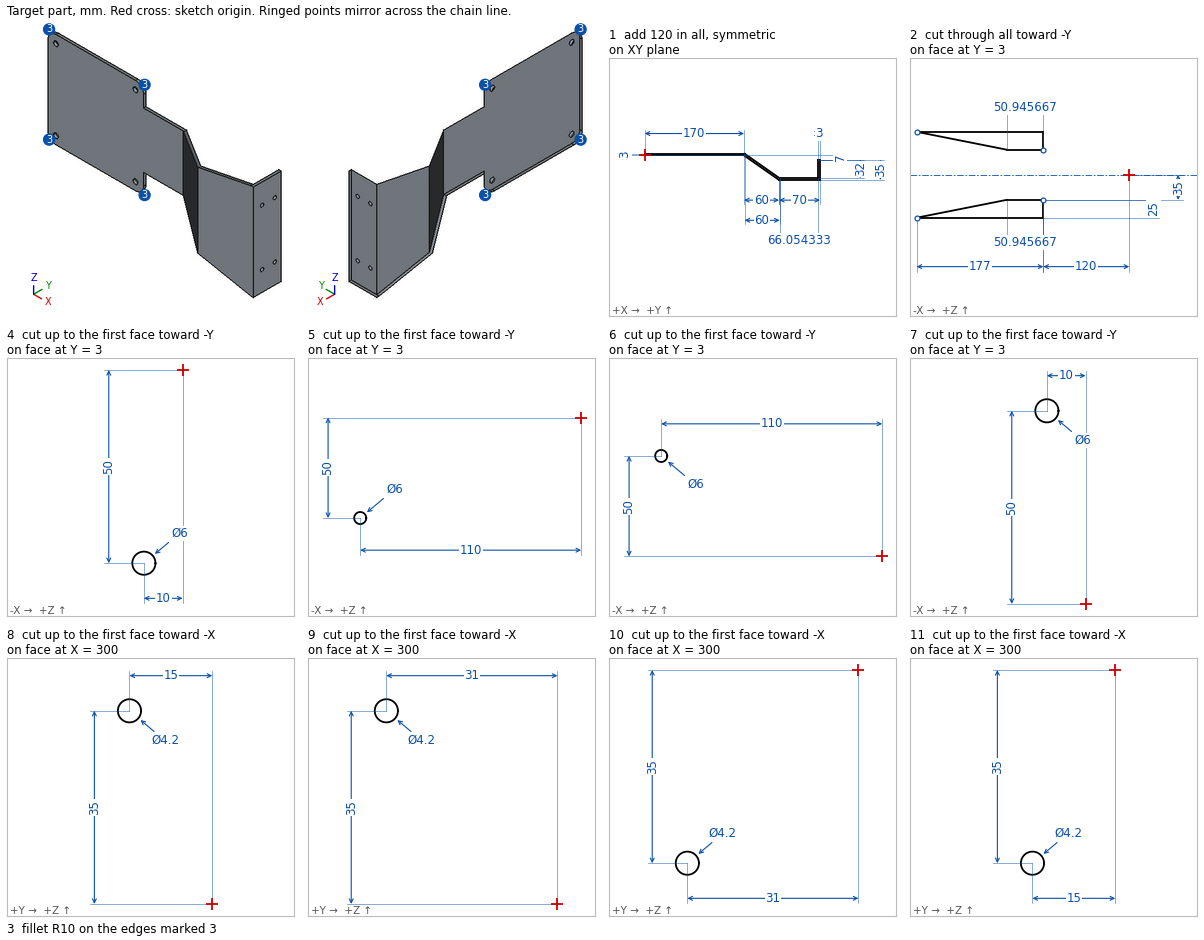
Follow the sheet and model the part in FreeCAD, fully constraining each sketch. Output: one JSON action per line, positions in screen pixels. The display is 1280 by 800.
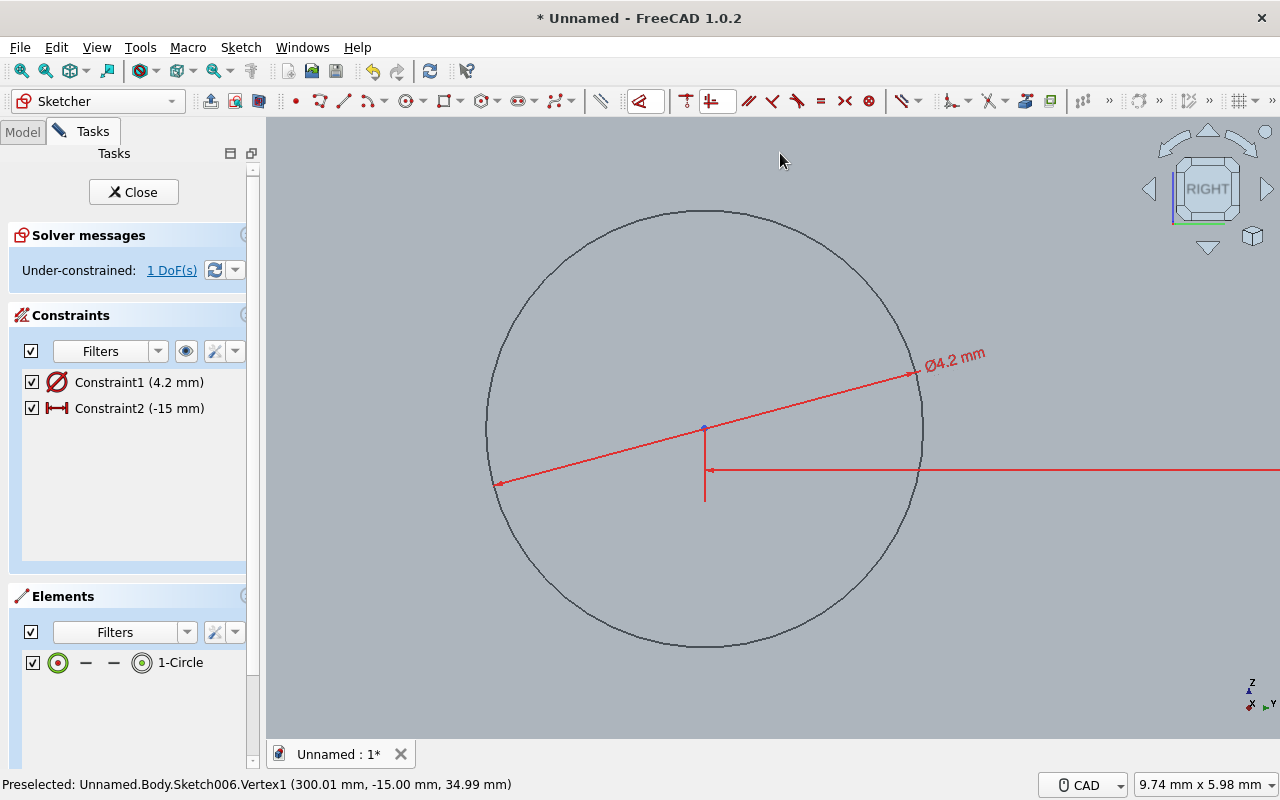
{"action": "left_click", "coordinate": [705, 429]}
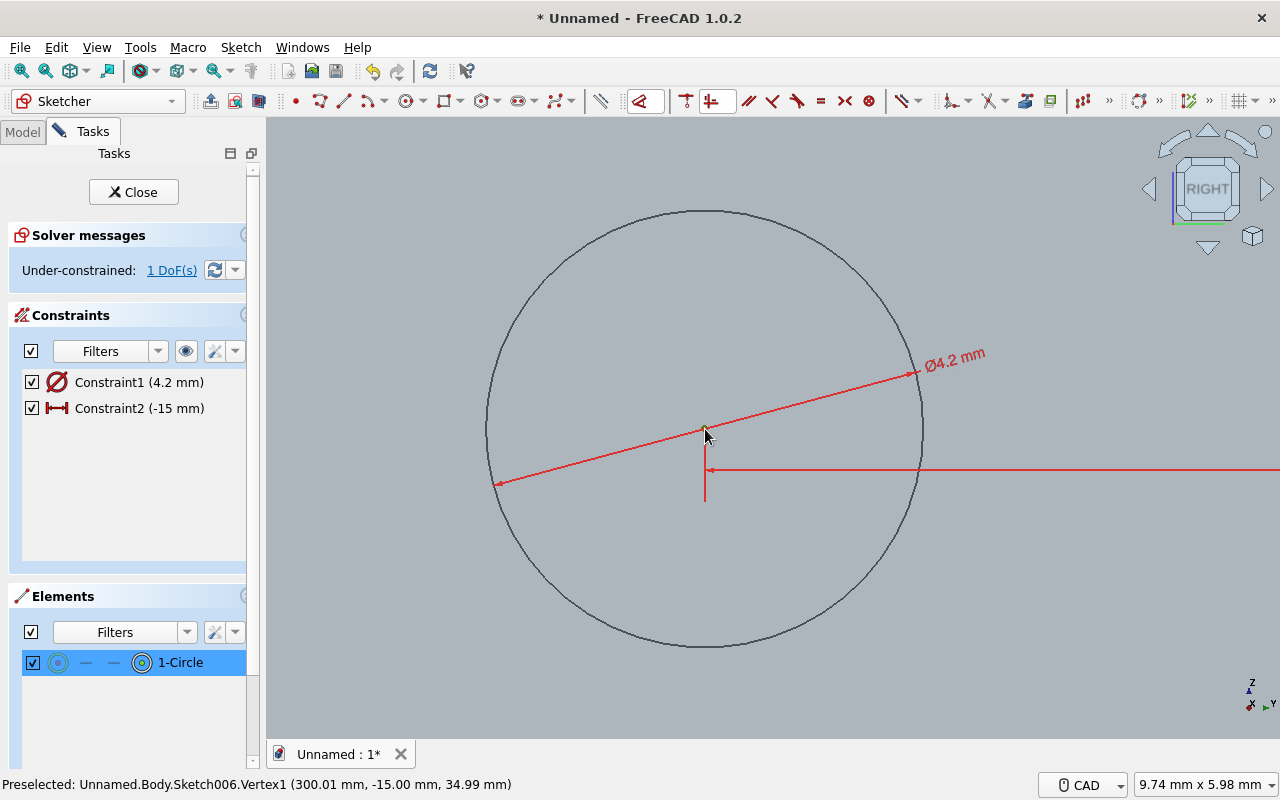
{"action": "left_click", "coordinate": [658, 102]}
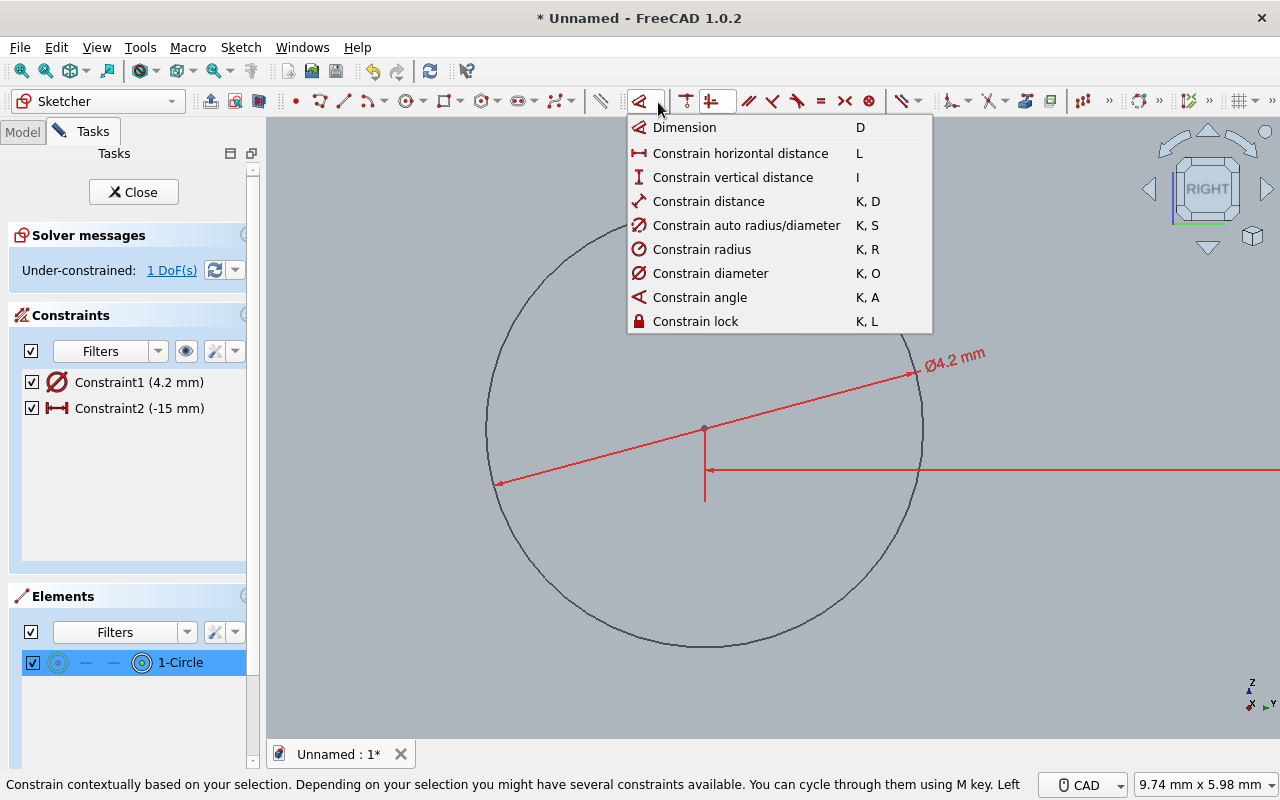
{"action": "left_click", "coordinate": [780, 177]}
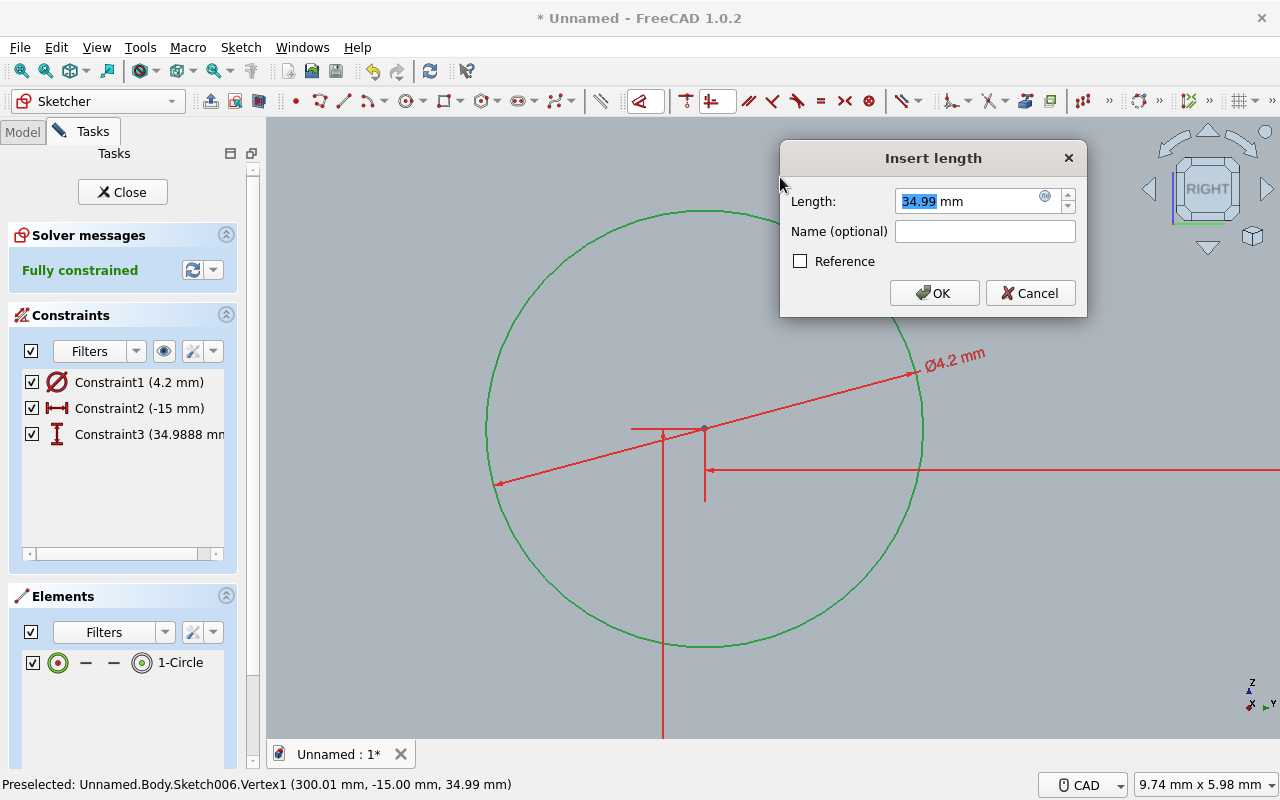
{"action": "type", "text": "35"}
{"action": "key", "text": "Return"}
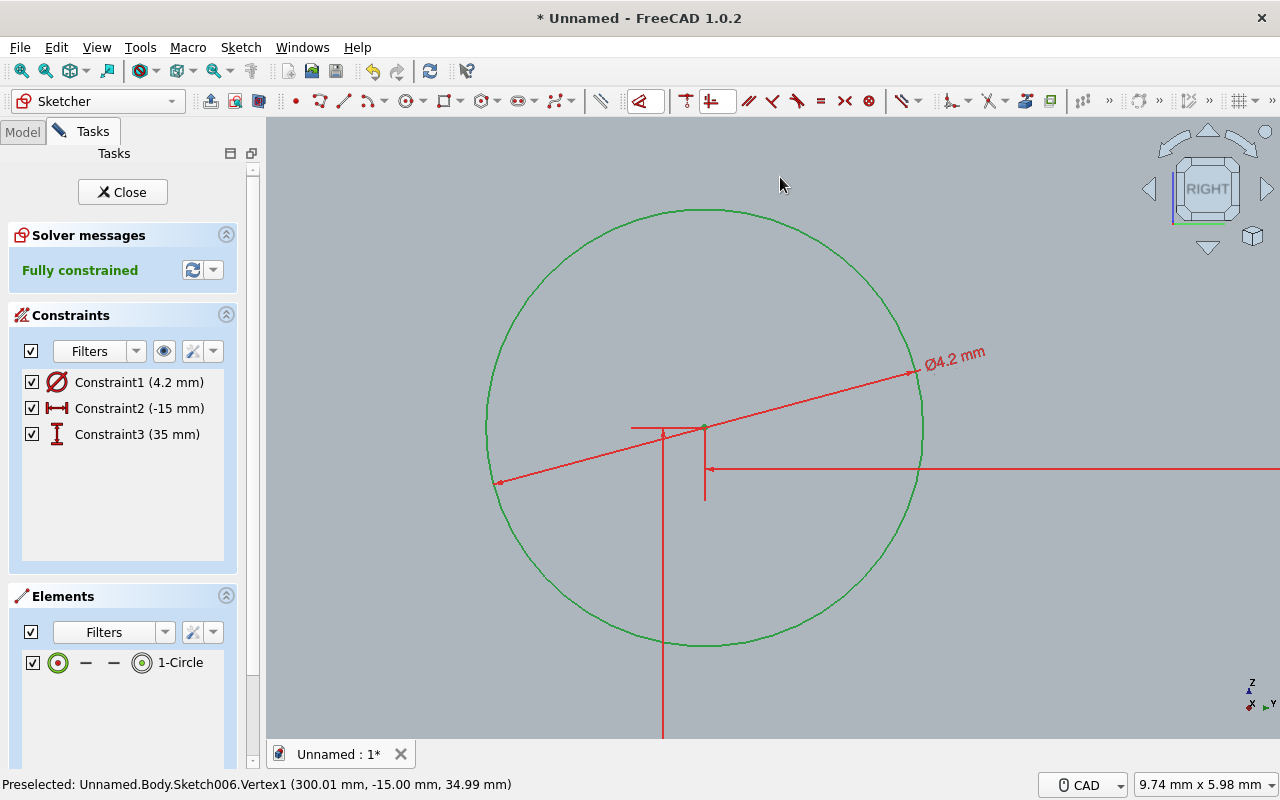
{"action": "left_click", "coordinate": [123, 192]}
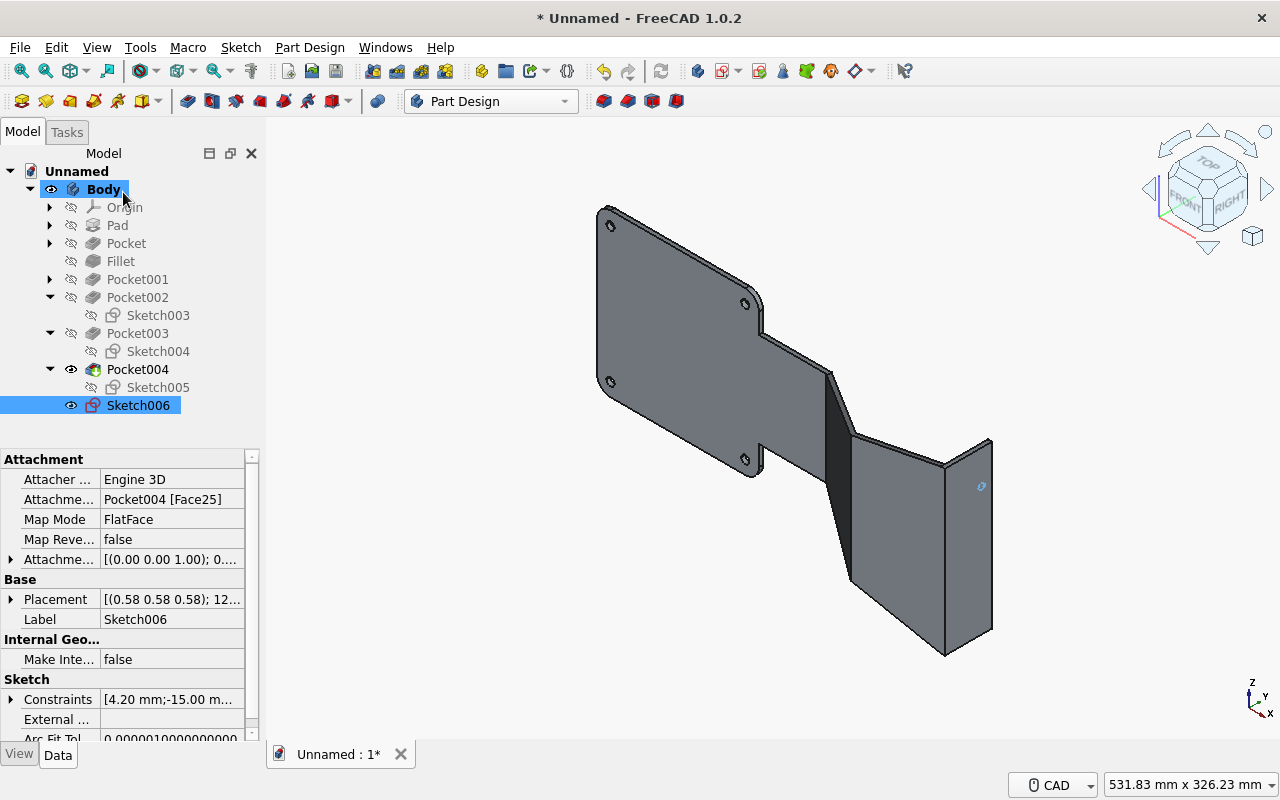
{"action": "left_click", "coordinate": [188, 102]}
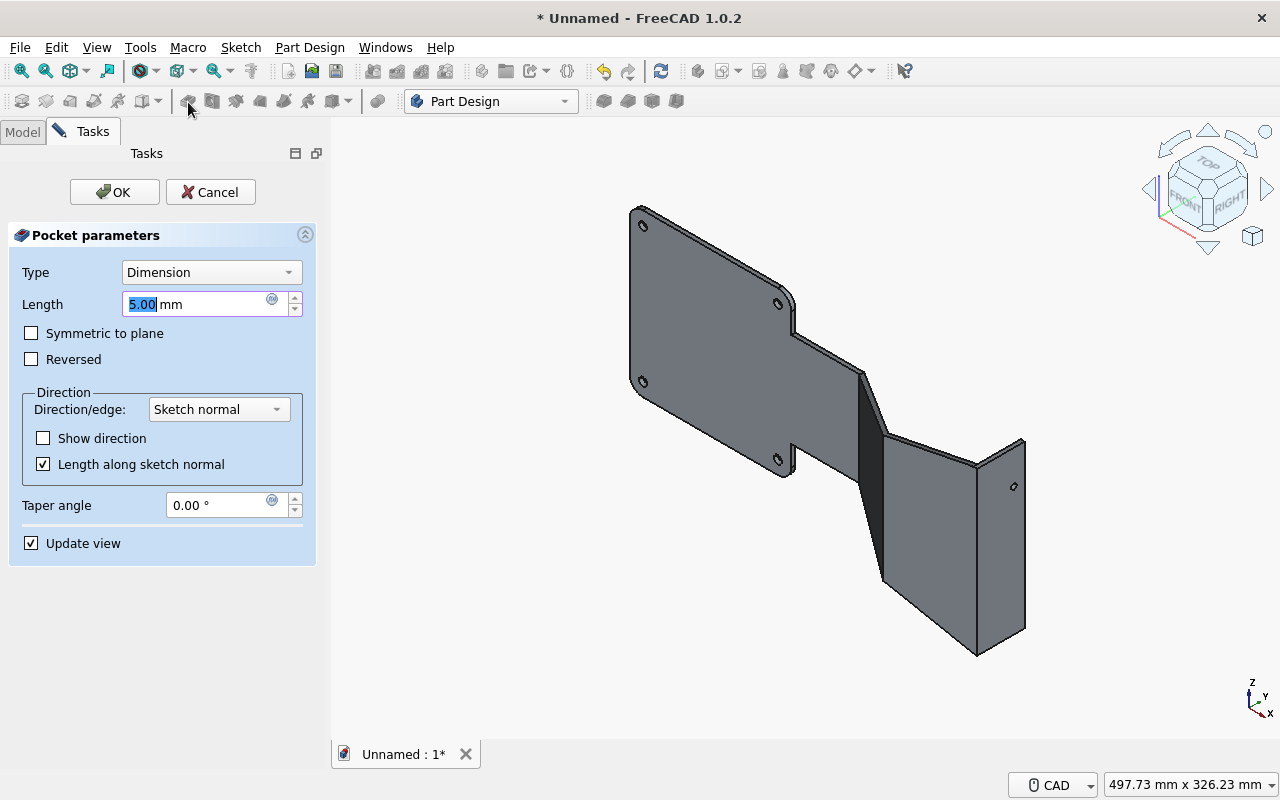
{"action": "left_click", "coordinate": [212, 272]}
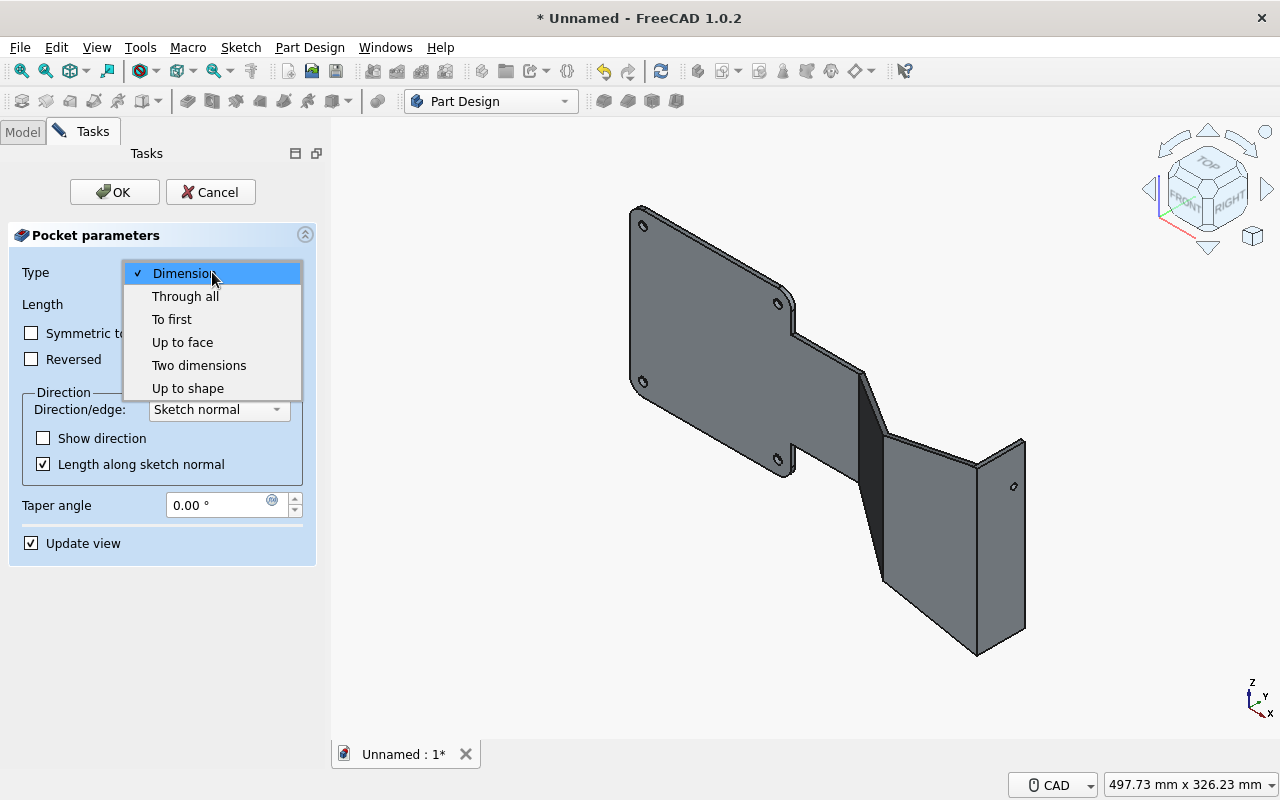
{"action": "left_click", "coordinate": [212, 320]}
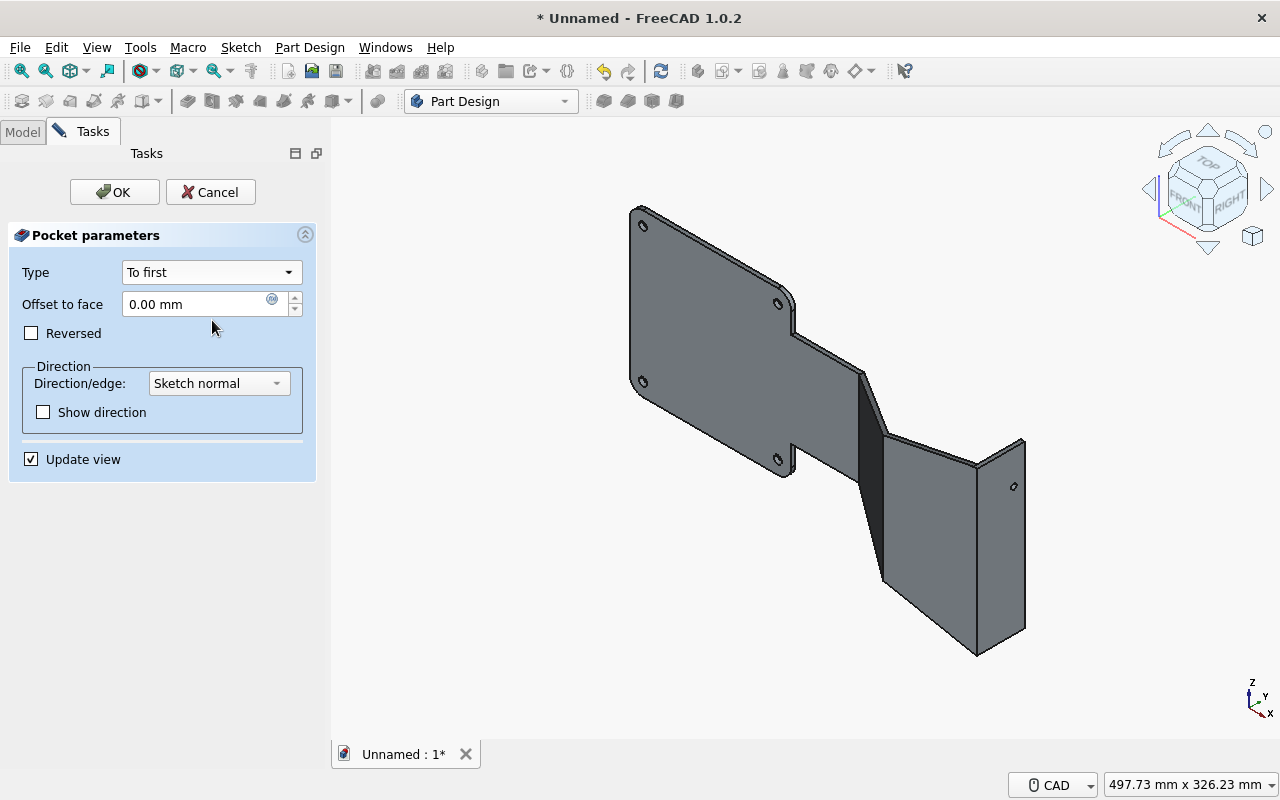
{"action": "left_click", "coordinate": [115, 192]}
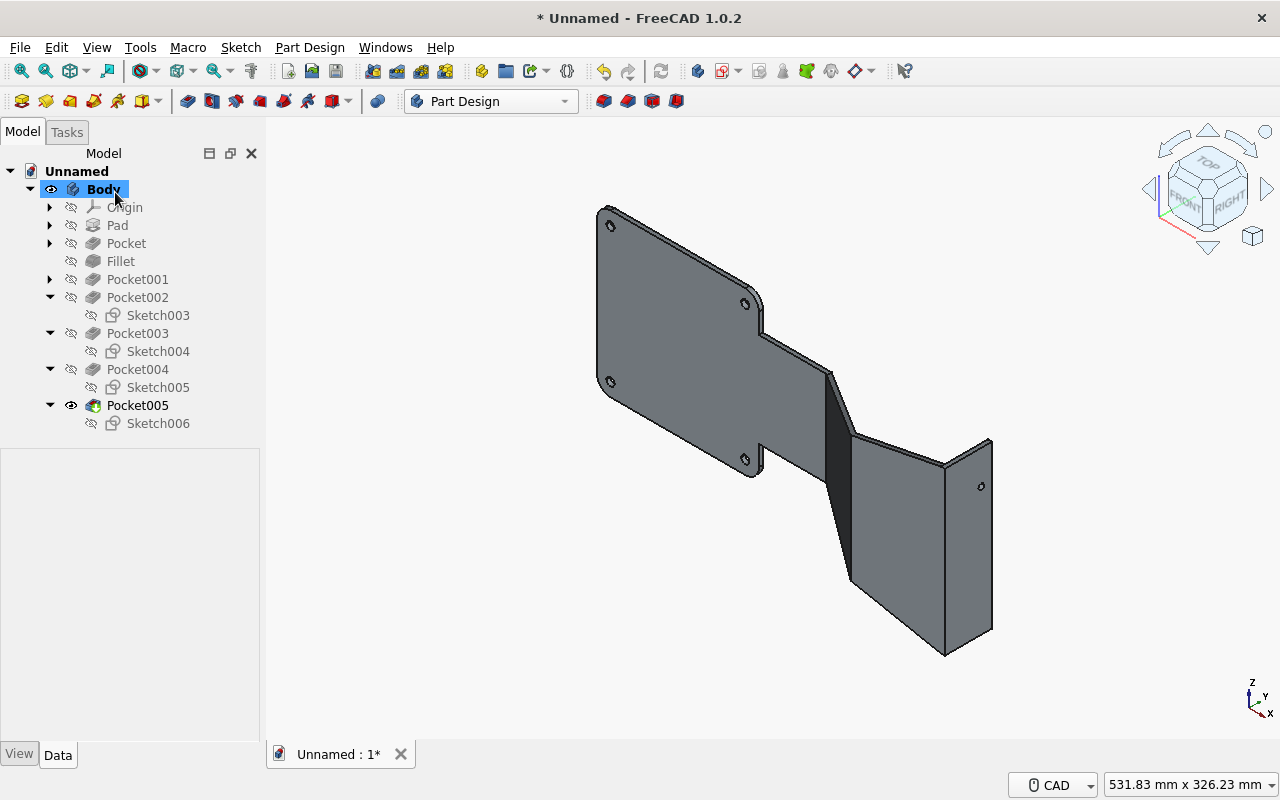
{"action": "left_click", "coordinate": [968, 521]}